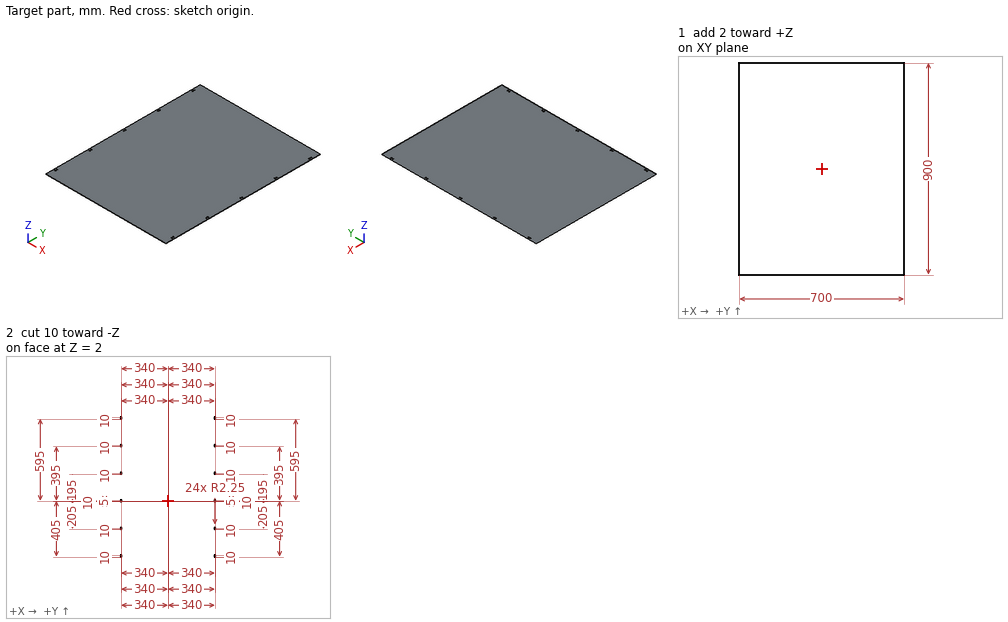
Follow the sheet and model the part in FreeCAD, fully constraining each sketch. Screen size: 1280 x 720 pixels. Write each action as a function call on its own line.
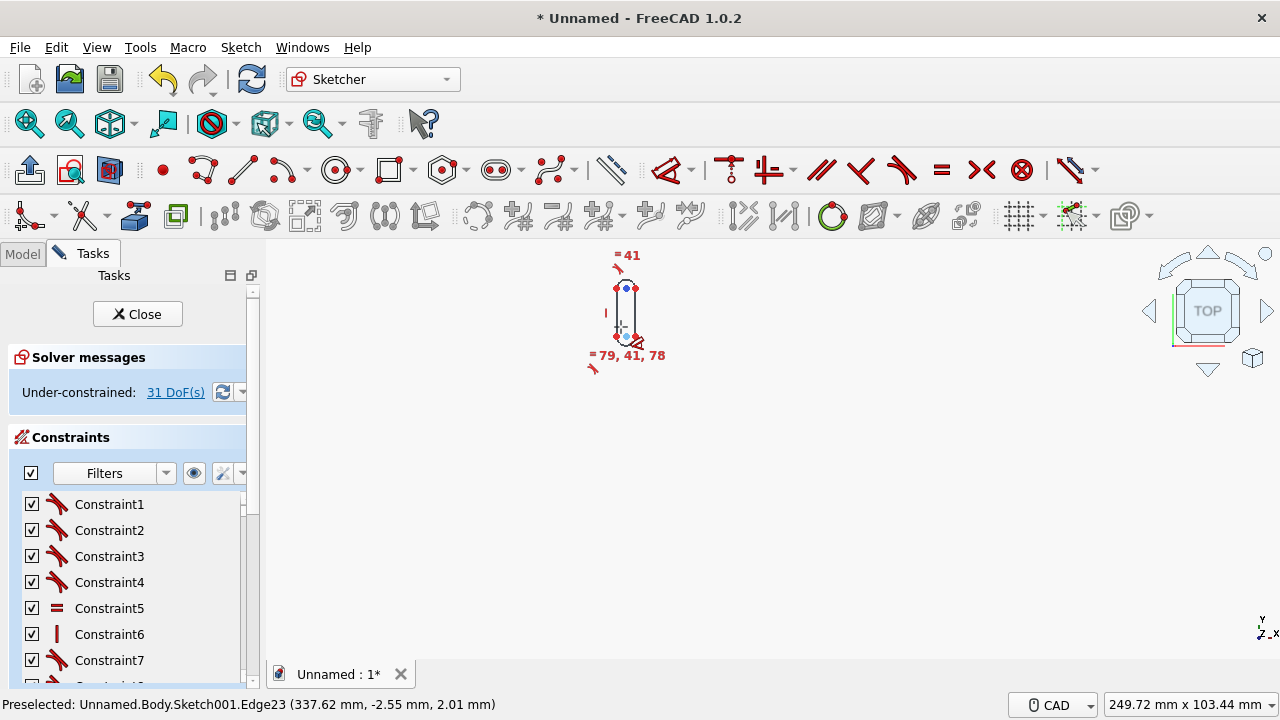
click(617, 322)
click(583, 313)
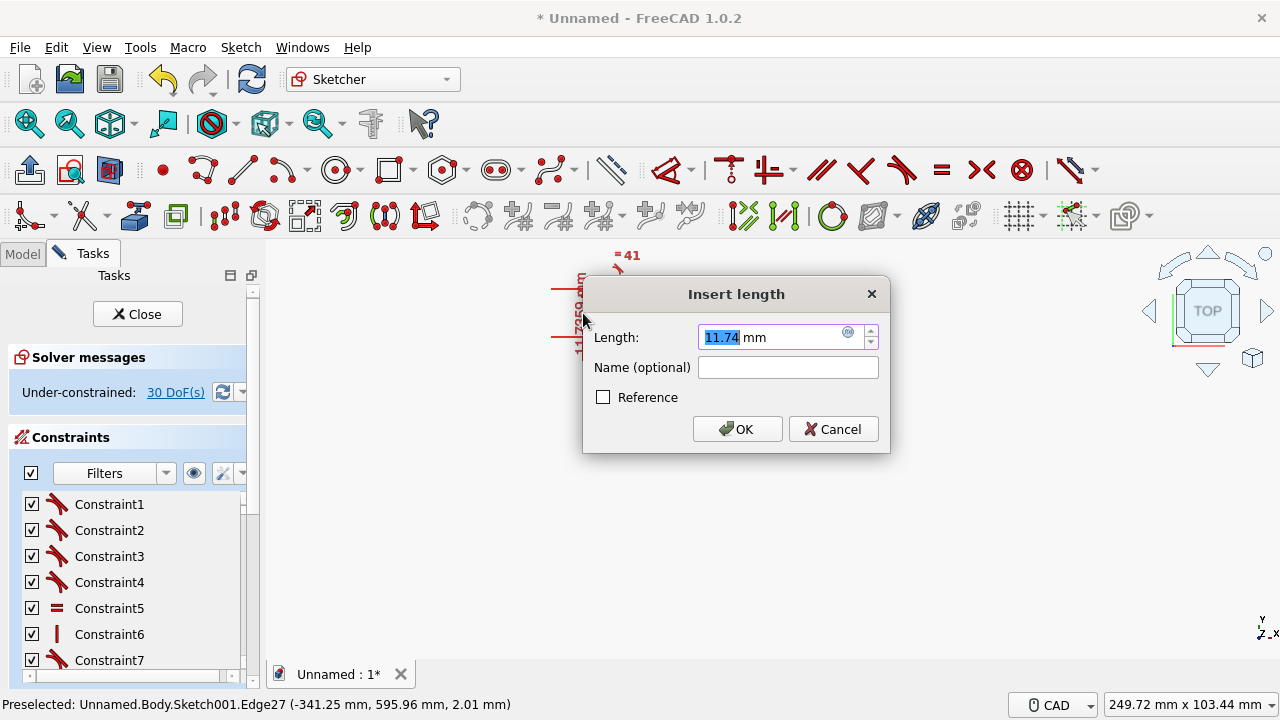
text(10)
key(Return)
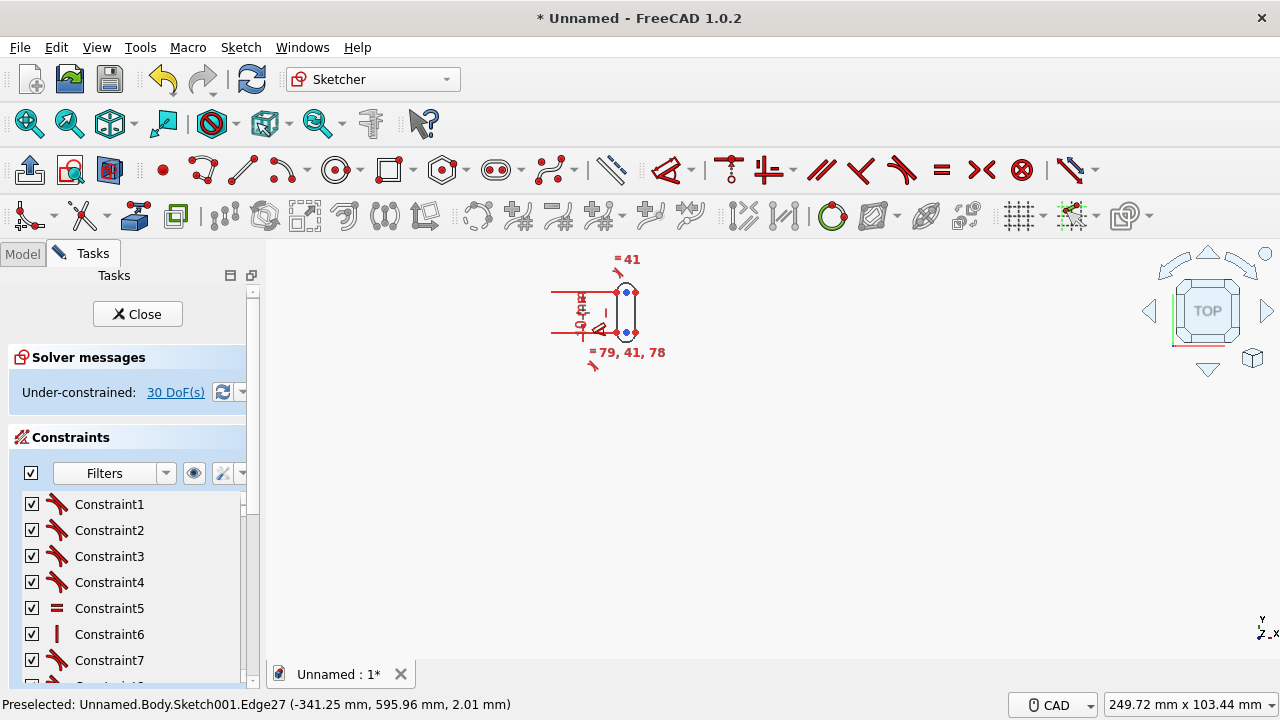
scroll(620, 327, down, 14)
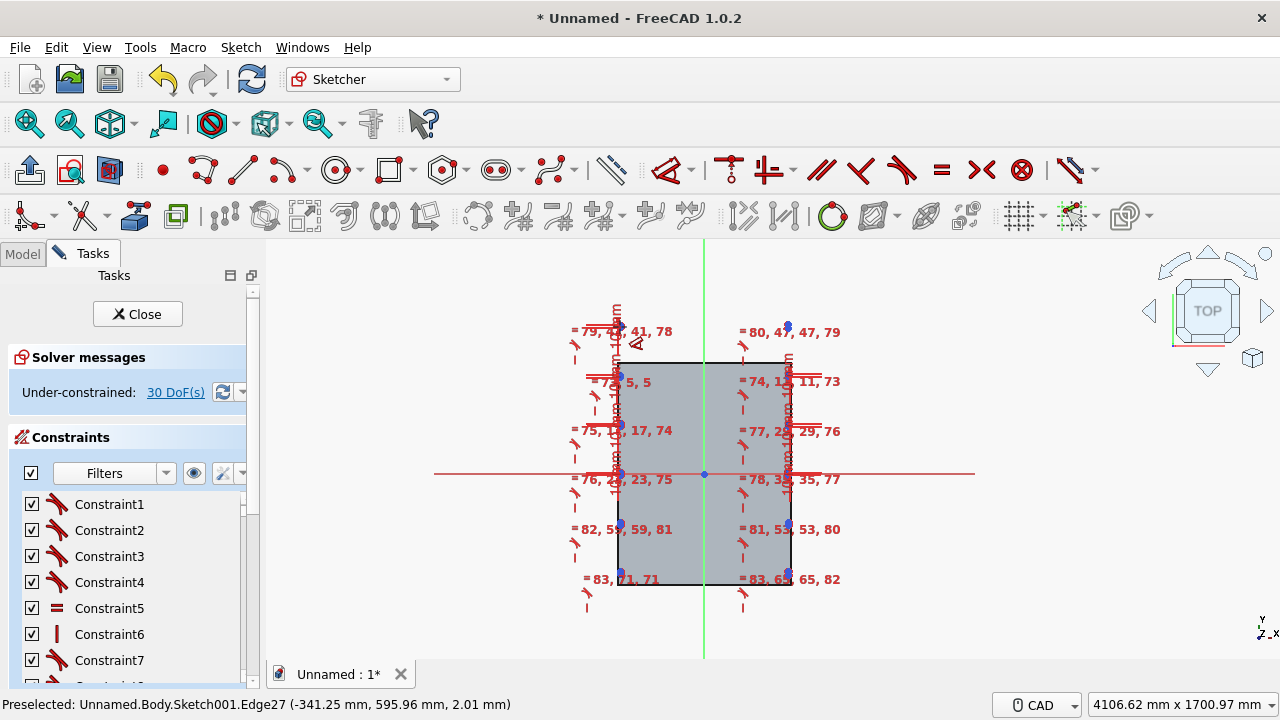
scroll(788, 327, up, 14)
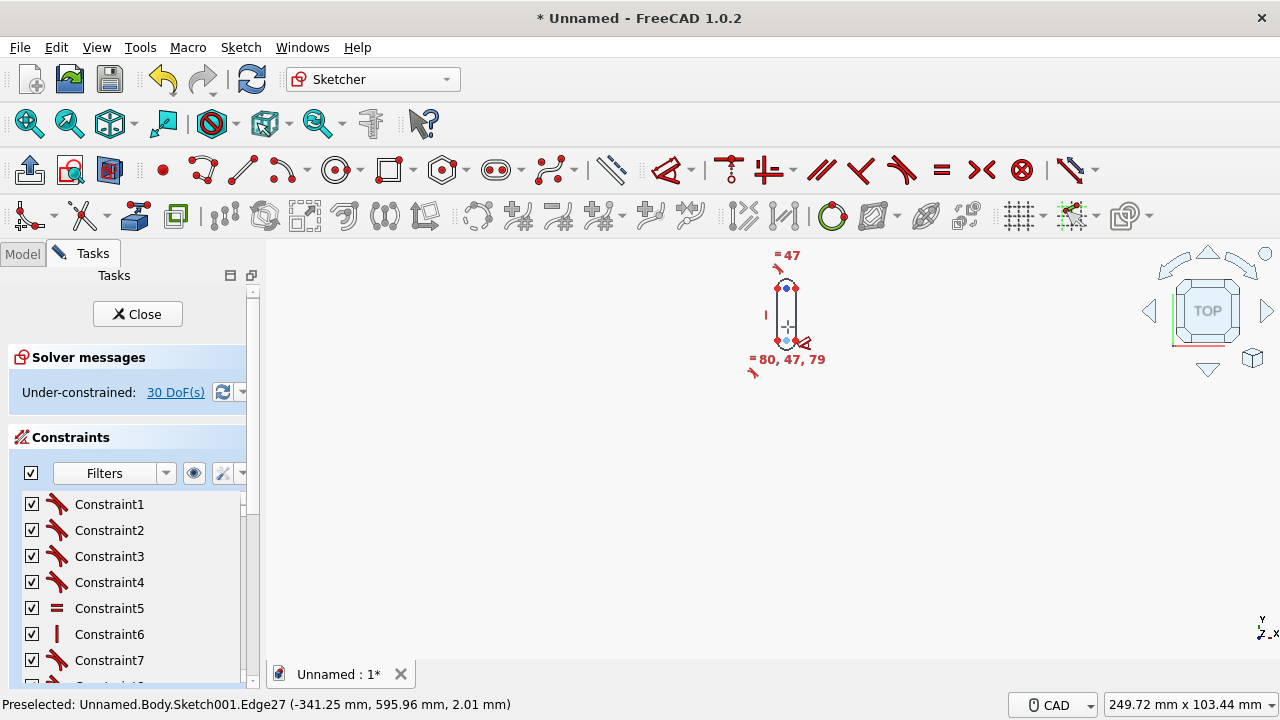
click(777, 325)
click(811, 314)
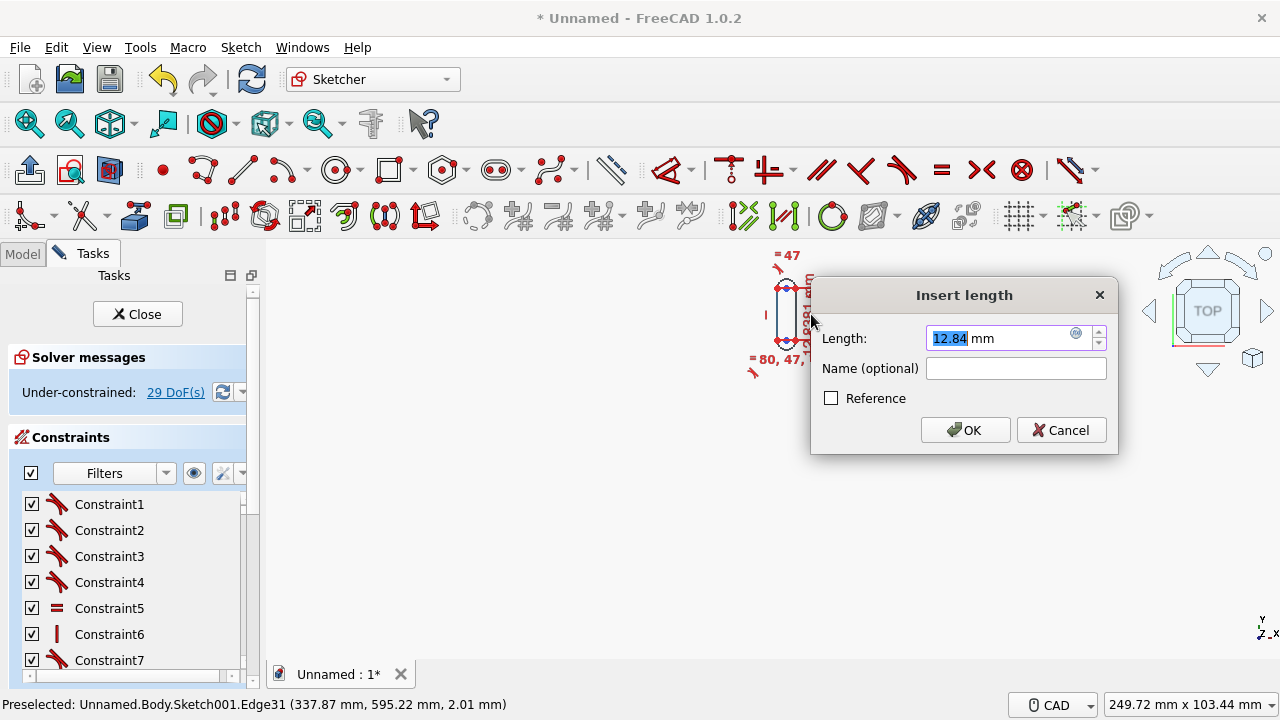
text(10)
key(Return)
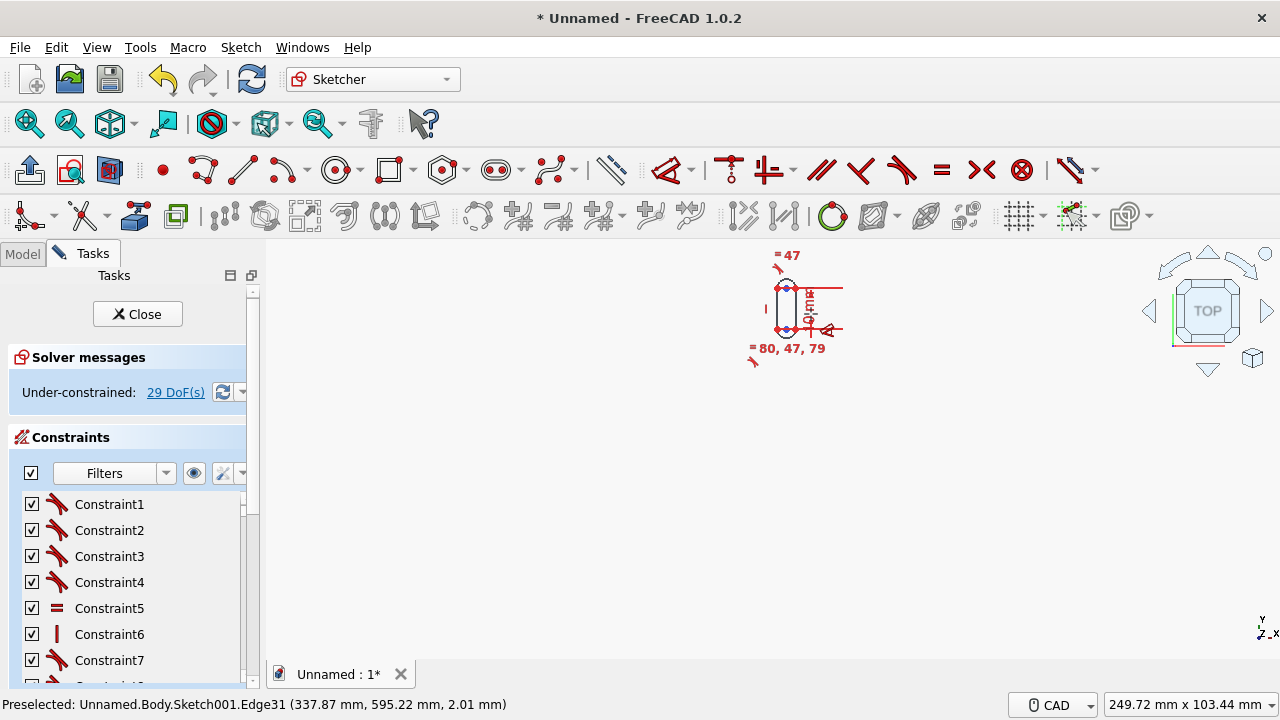
scroll(789, 327, down, 14)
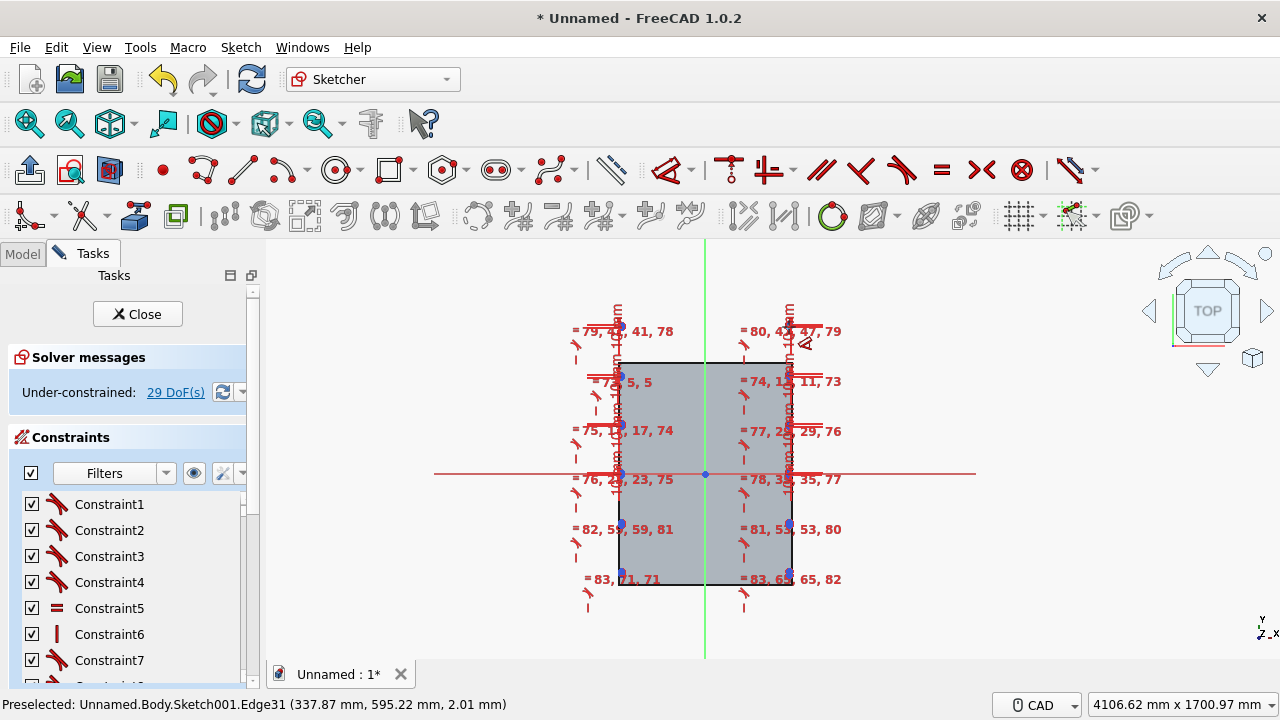
scroll(789, 524, up, 14)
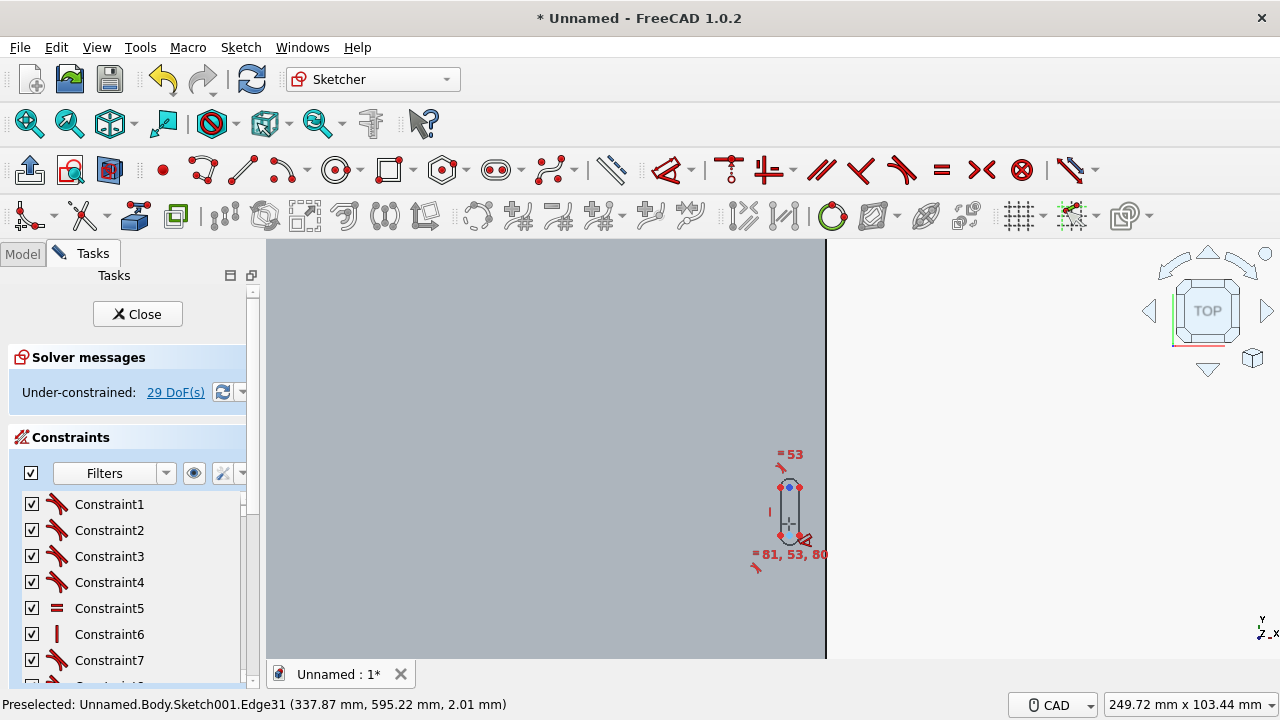
click(781, 521)
click(815, 512)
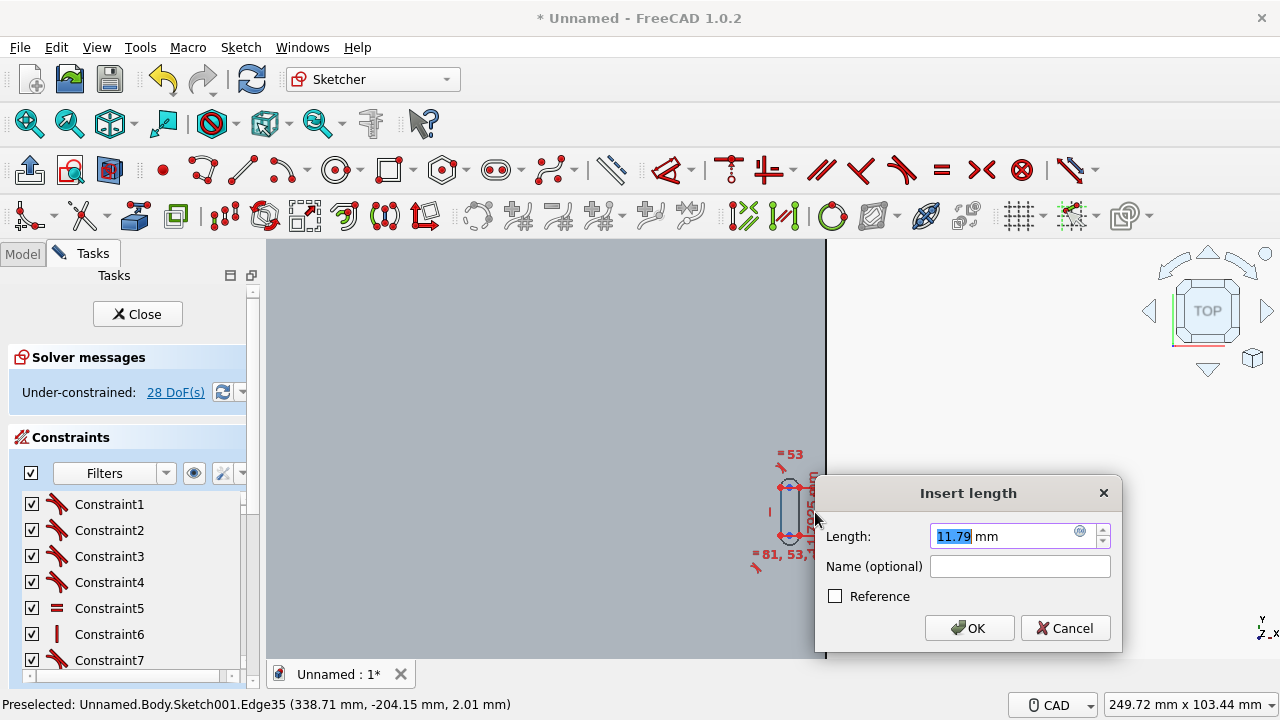
text(10)
key(Return)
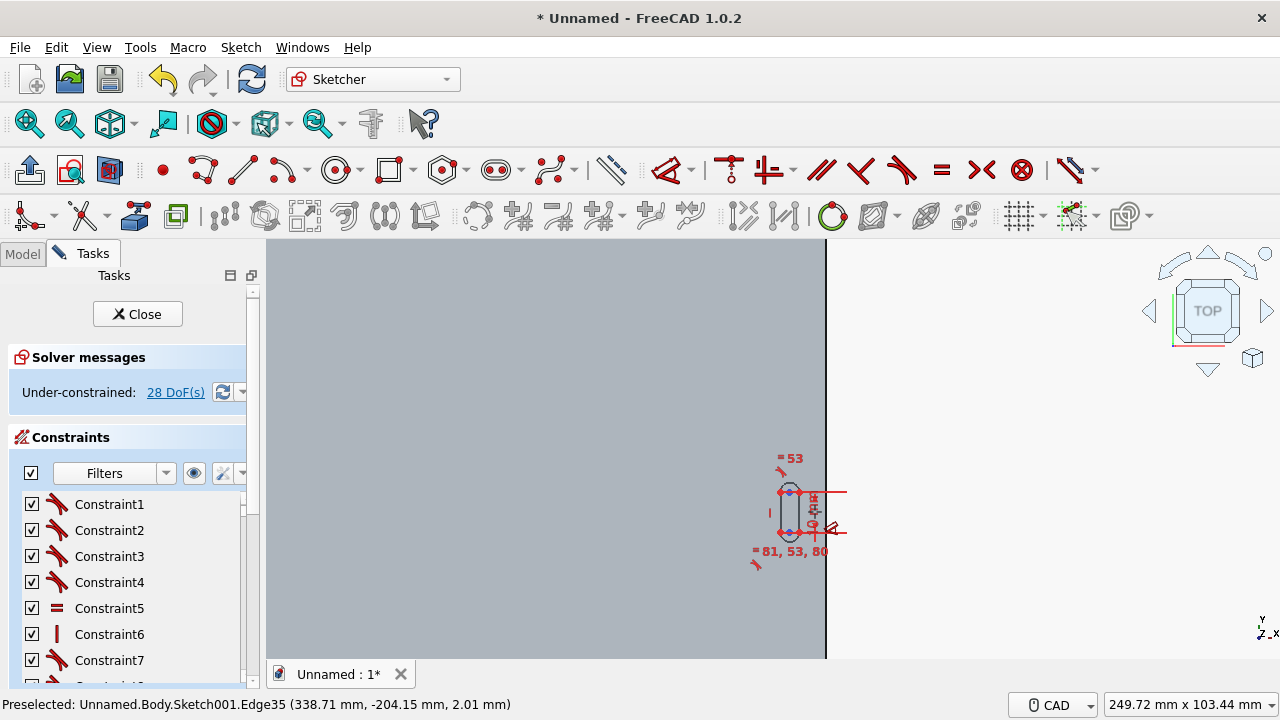
scroll(789, 524, down, 14)